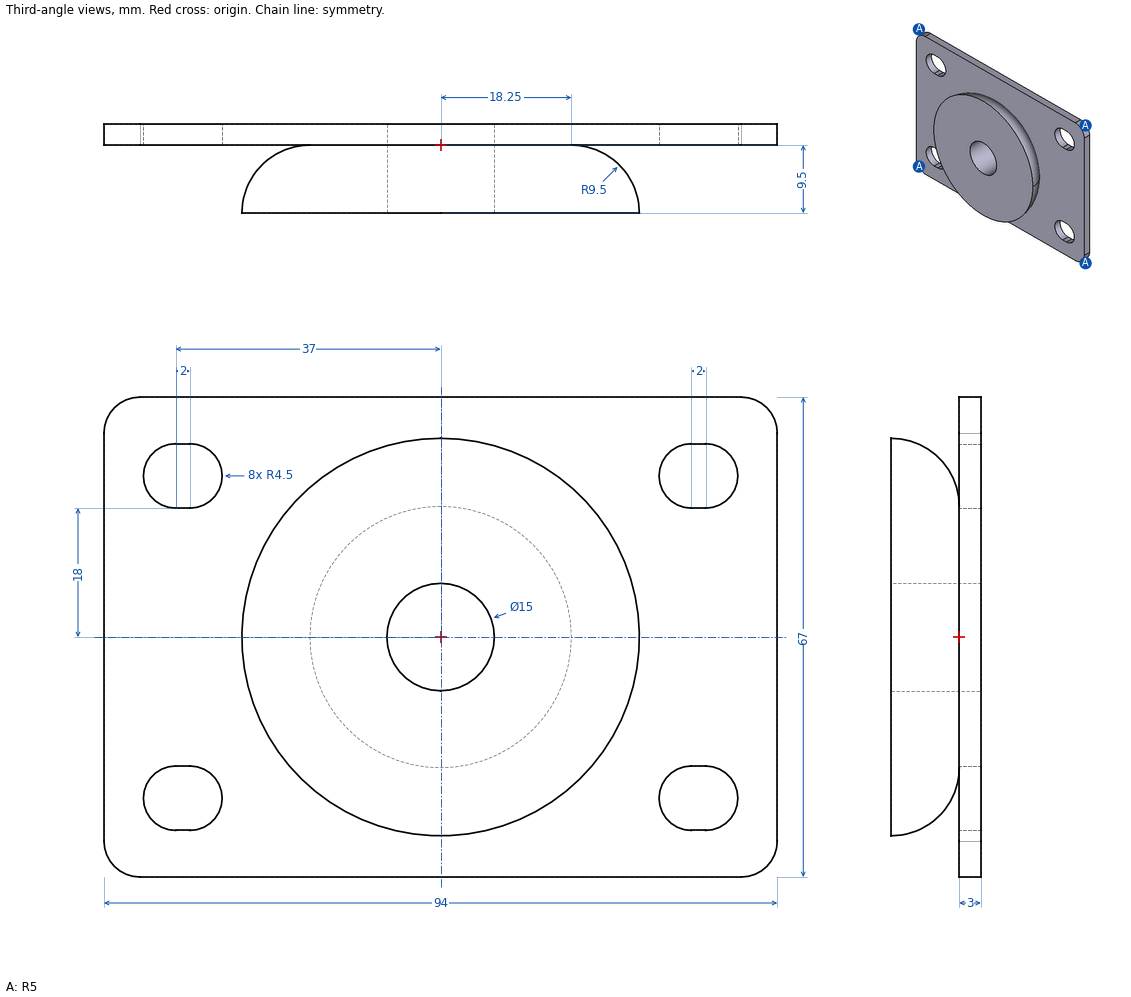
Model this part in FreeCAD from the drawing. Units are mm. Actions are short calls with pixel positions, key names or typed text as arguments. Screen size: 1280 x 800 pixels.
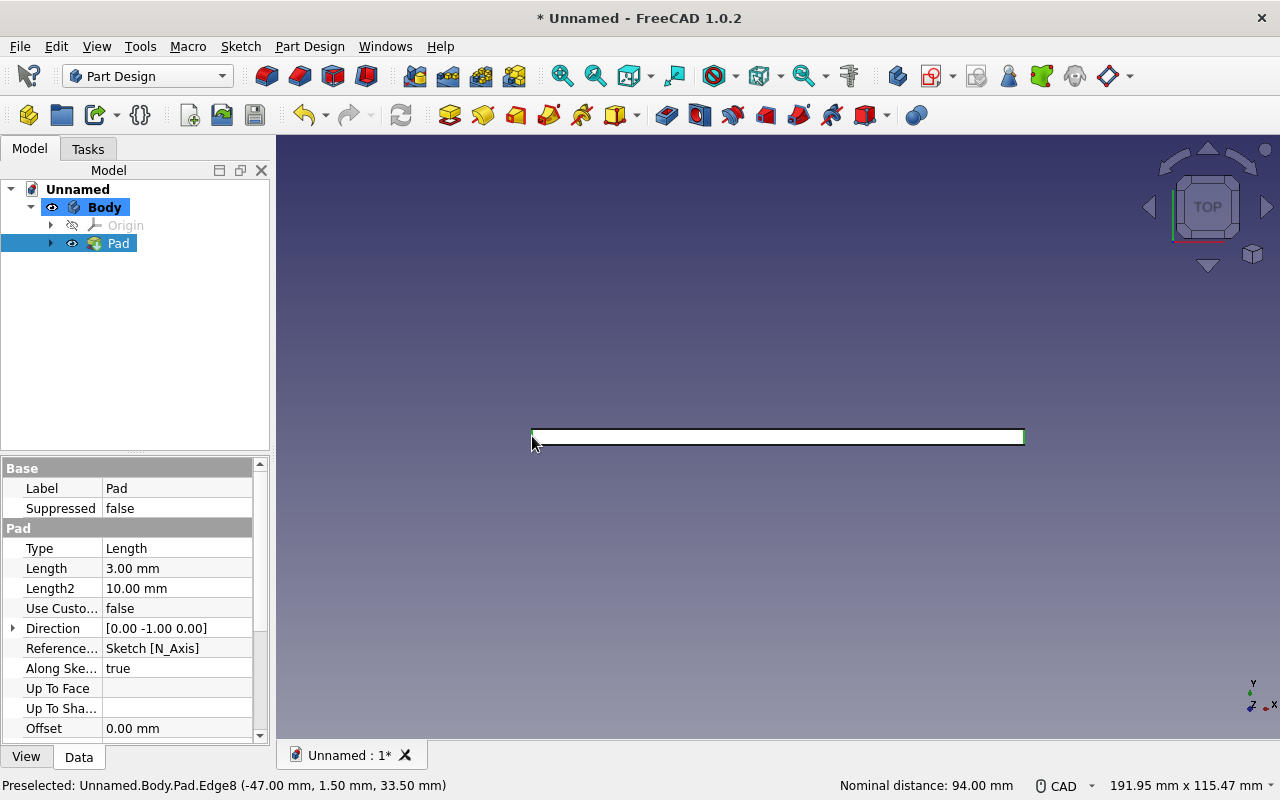
scroll(532, 436, up, 5)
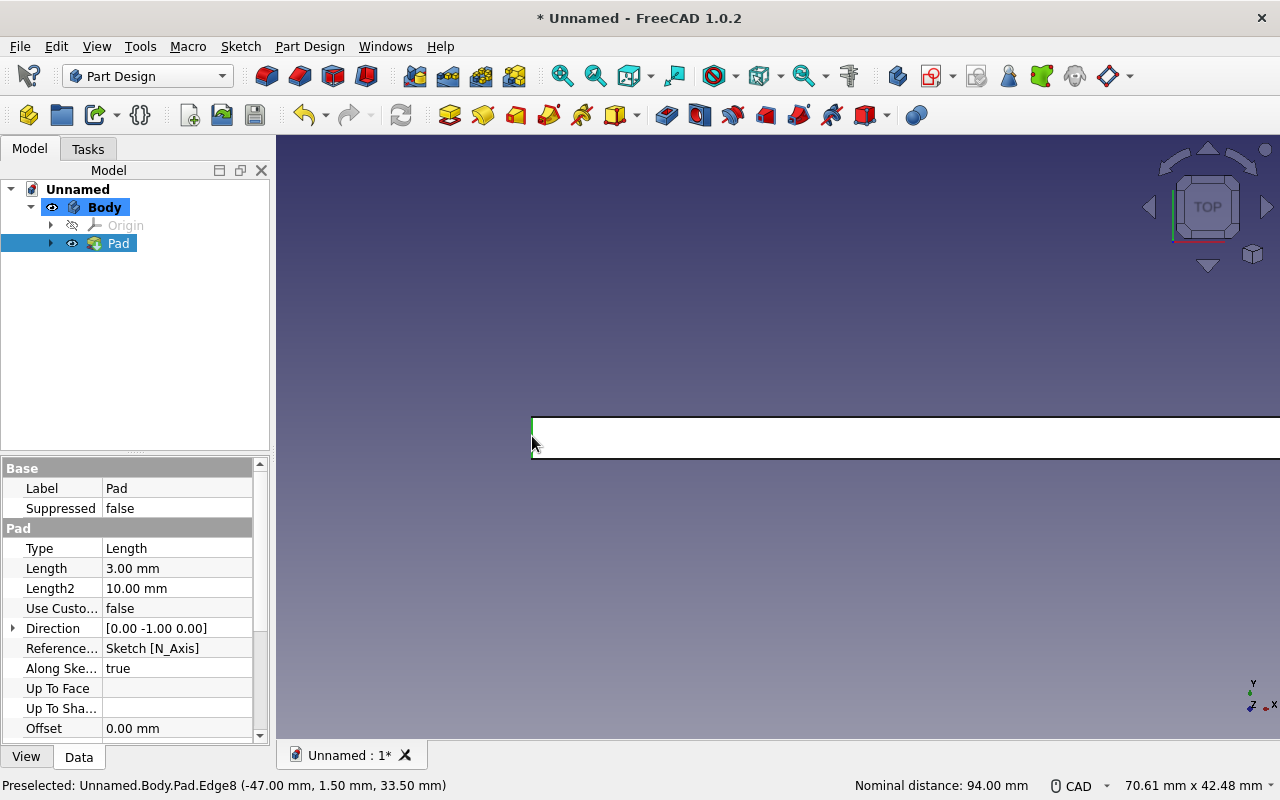
click(563, 76)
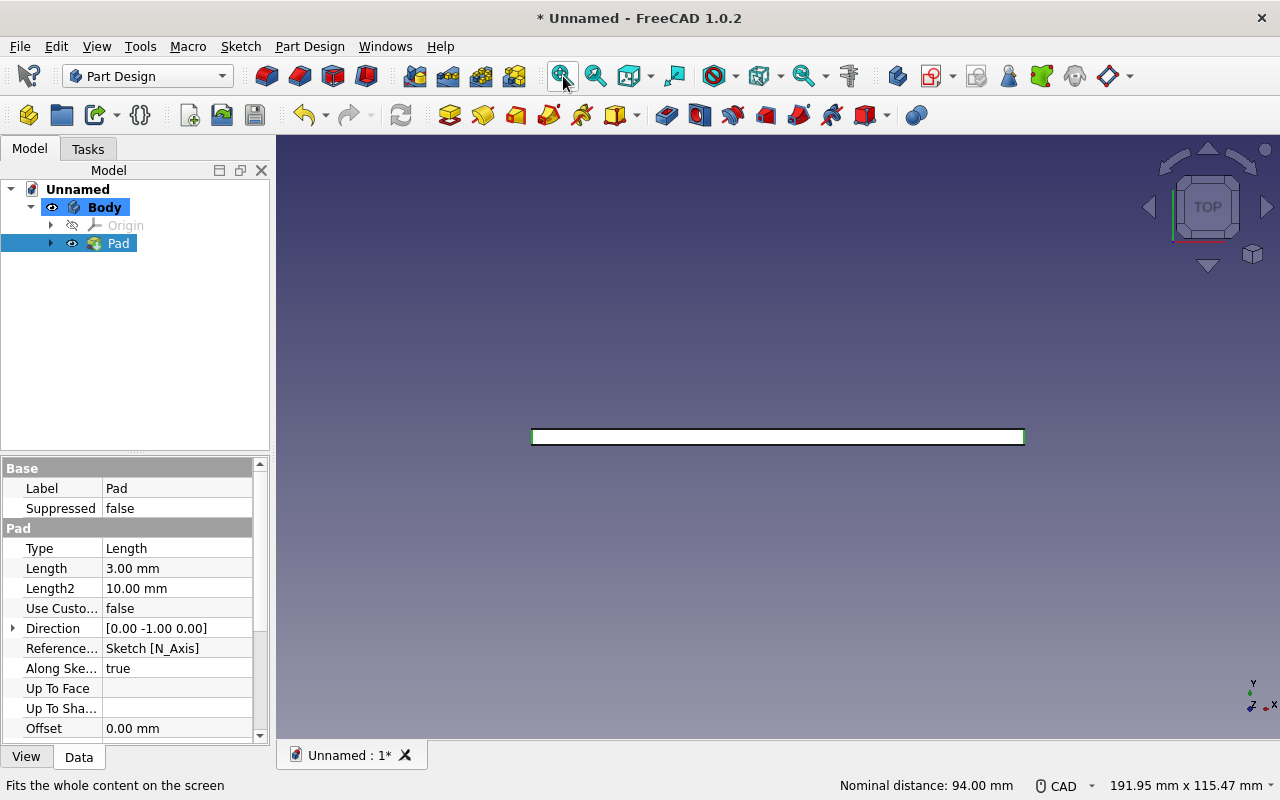
key(1)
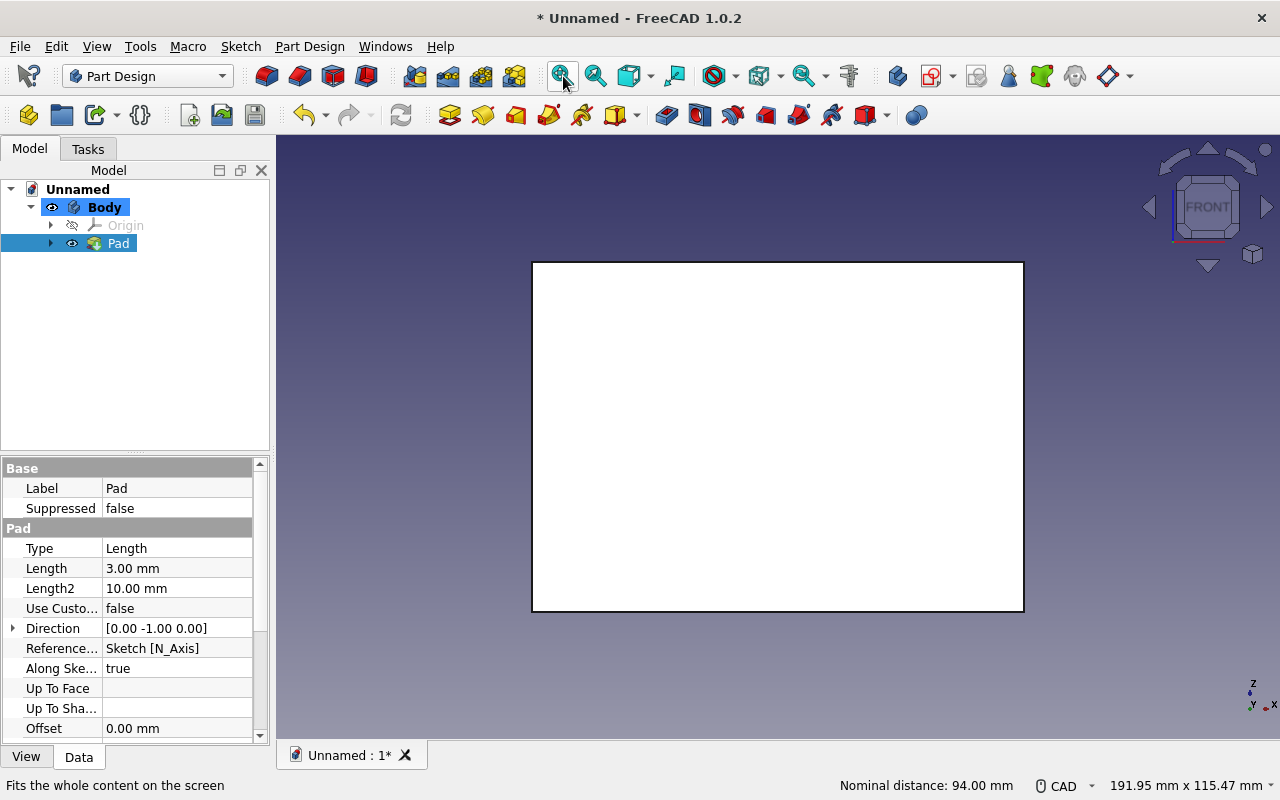
scroll(532, 611, up, 5)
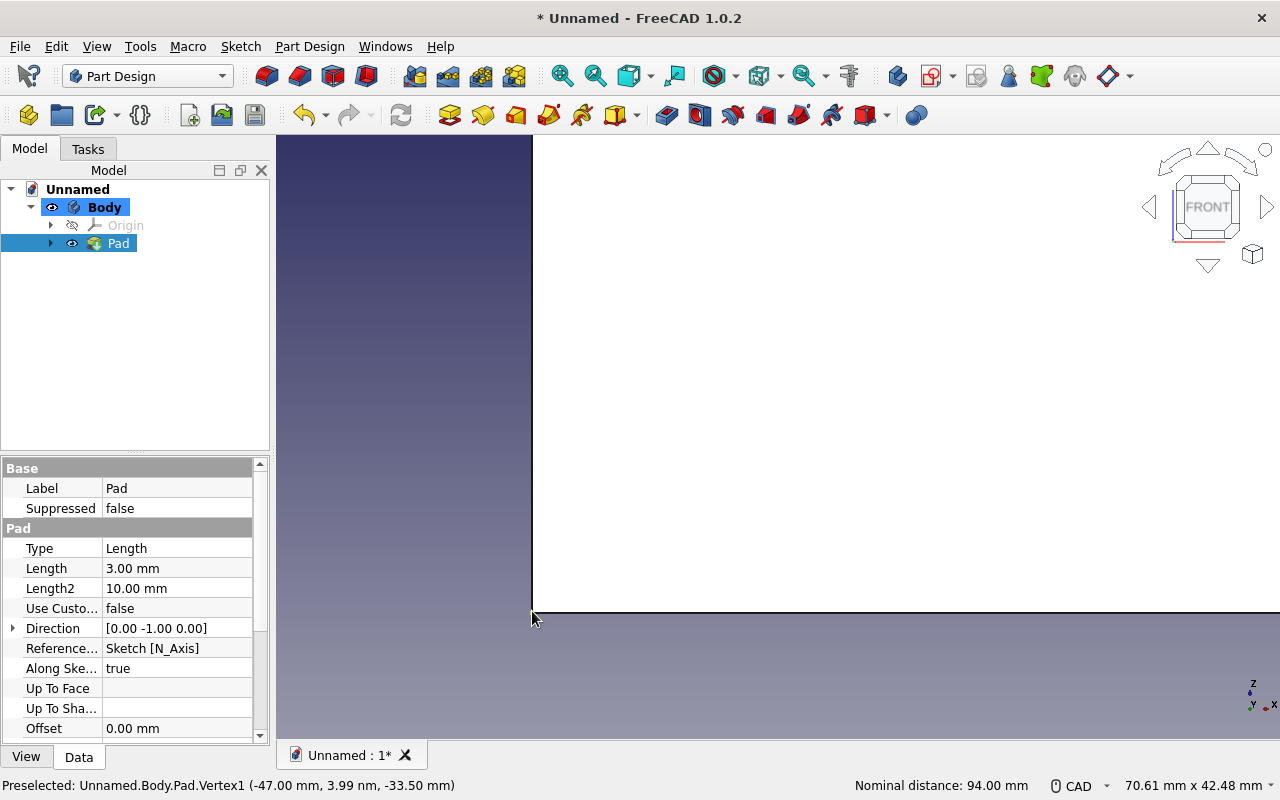
key(v)
key(f)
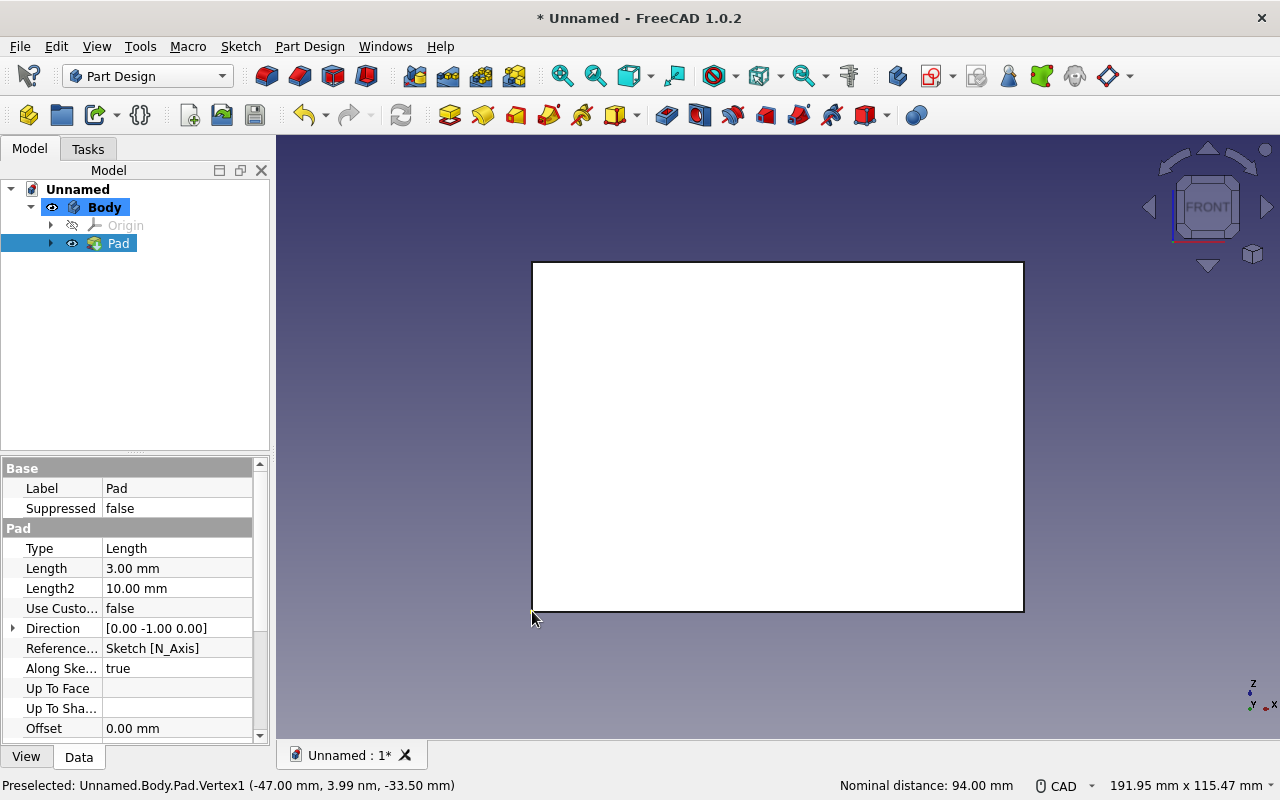
key(3)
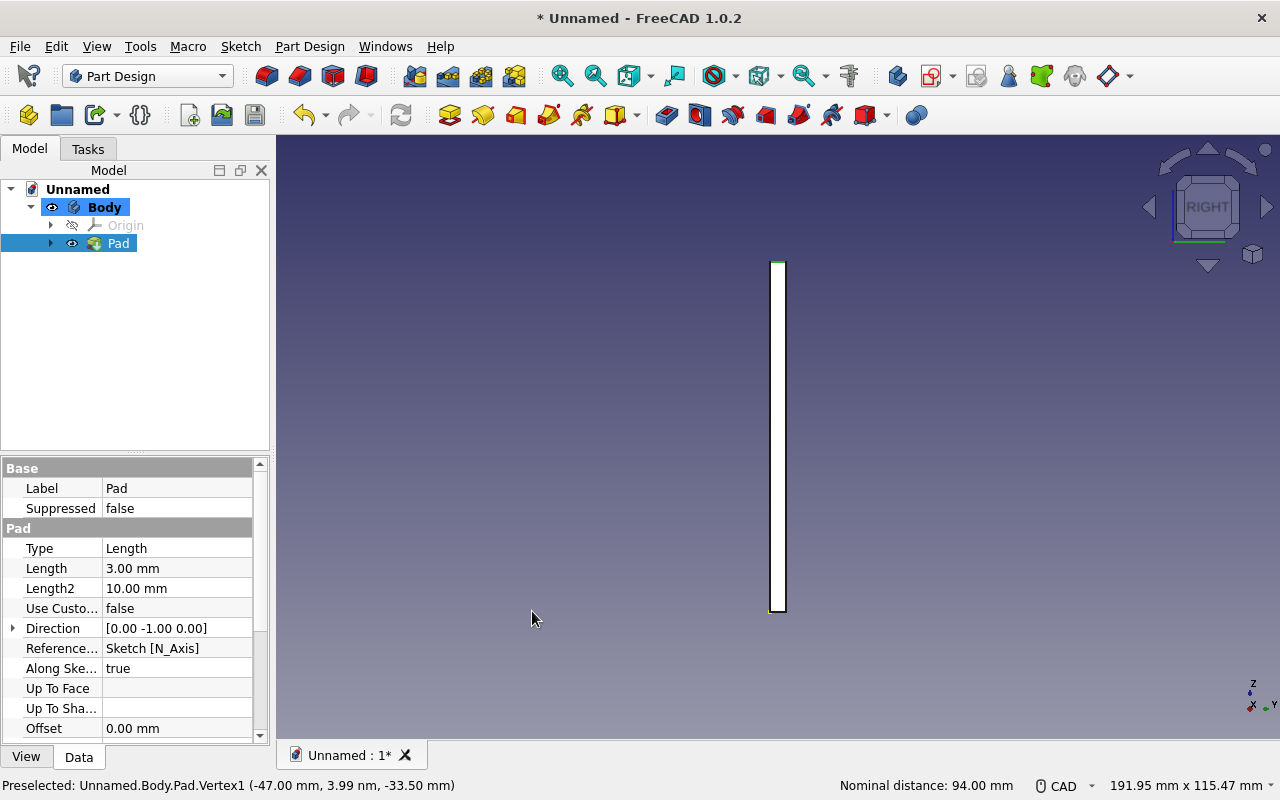
click(778, 611, ctrl)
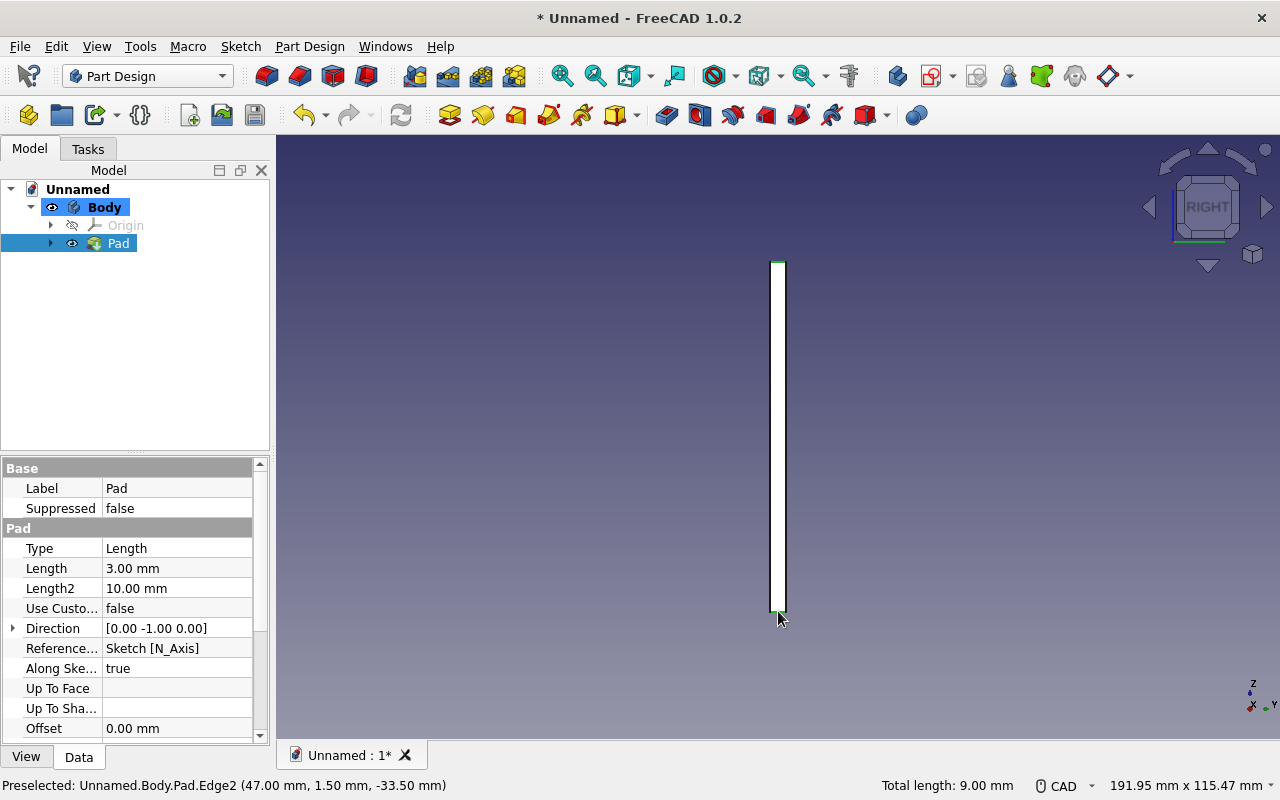
scroll(778, 611, up, 5)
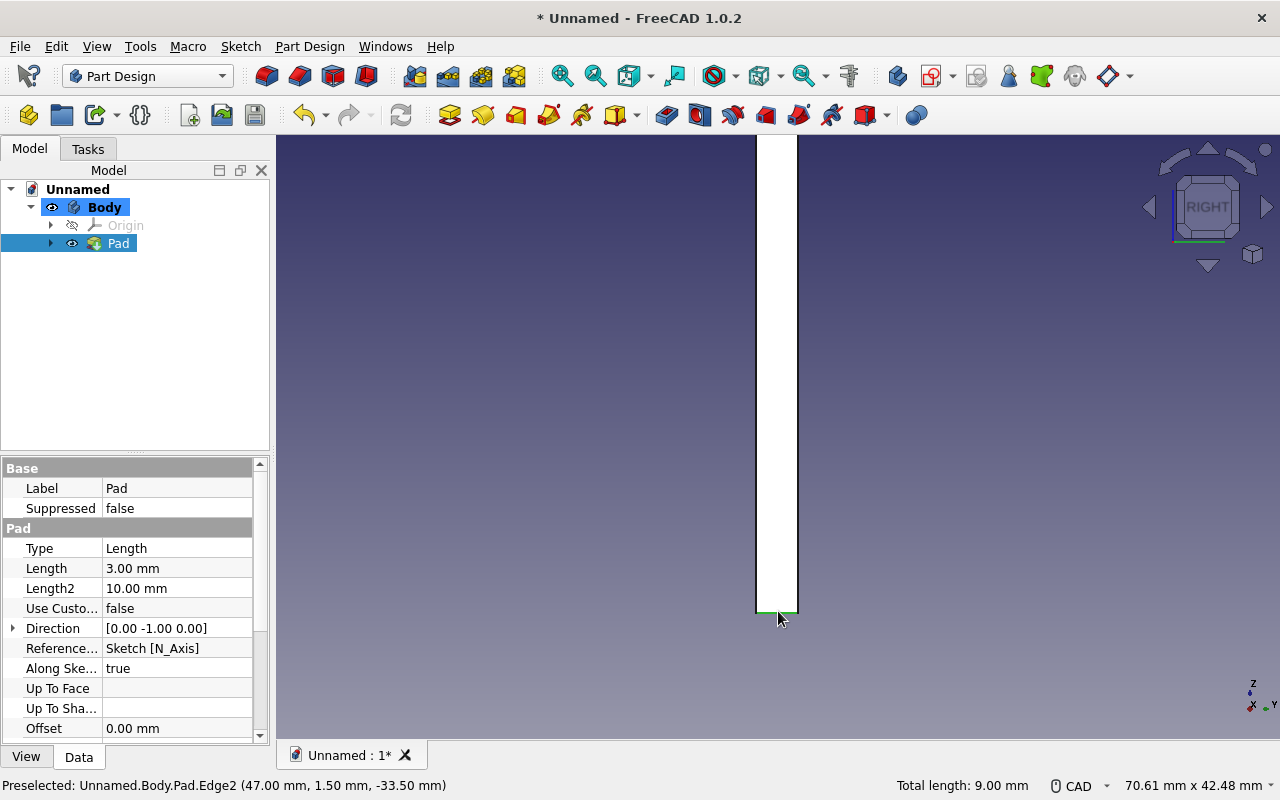
key(v)
key(f)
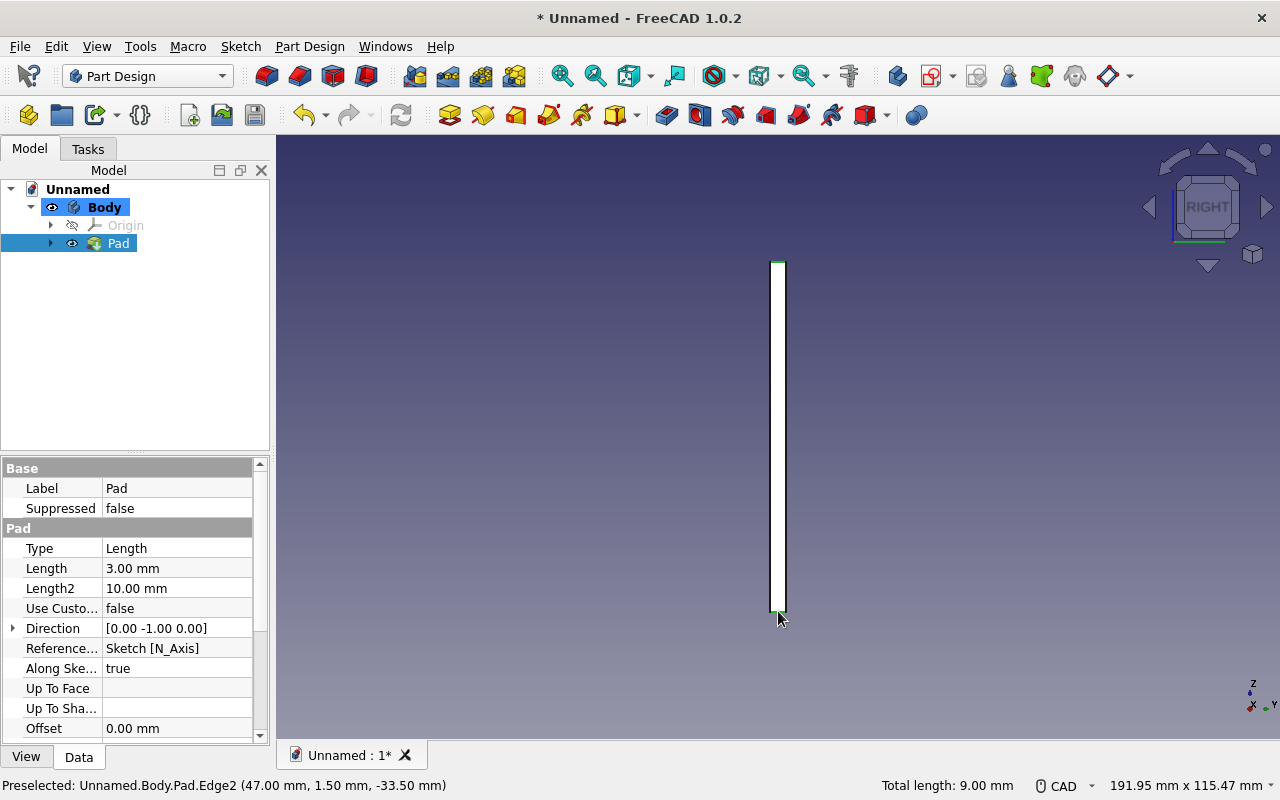
key(5)